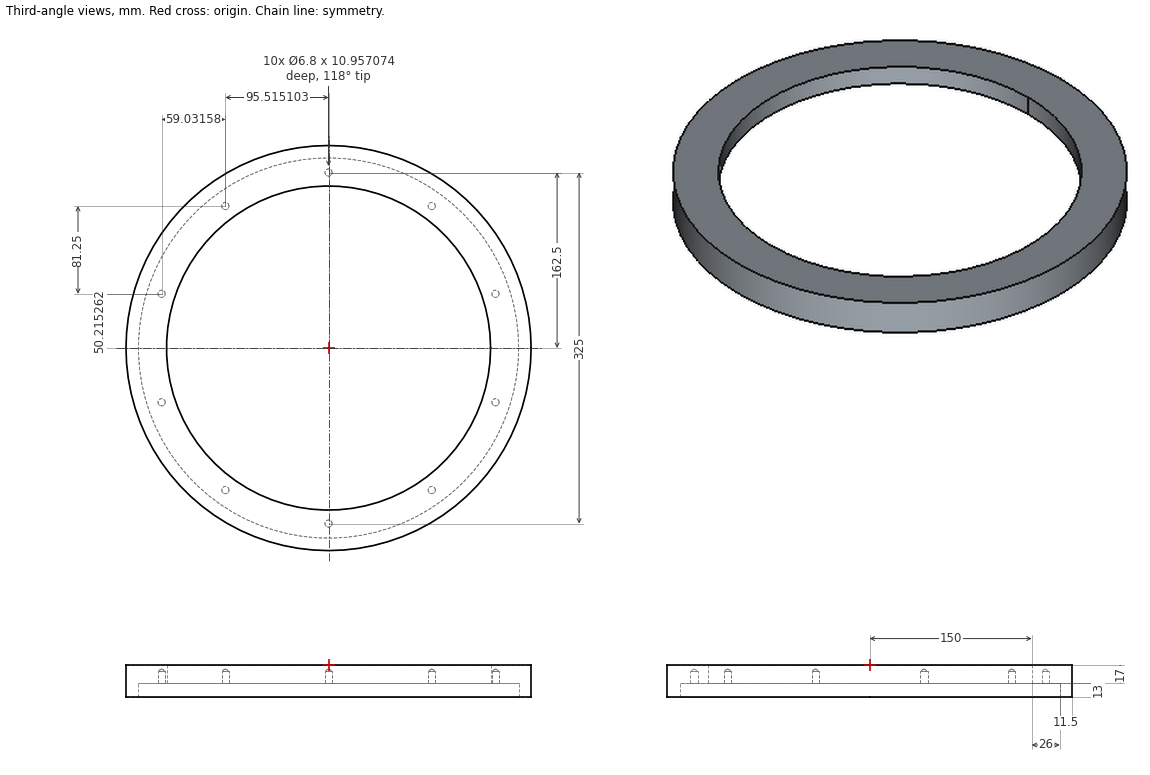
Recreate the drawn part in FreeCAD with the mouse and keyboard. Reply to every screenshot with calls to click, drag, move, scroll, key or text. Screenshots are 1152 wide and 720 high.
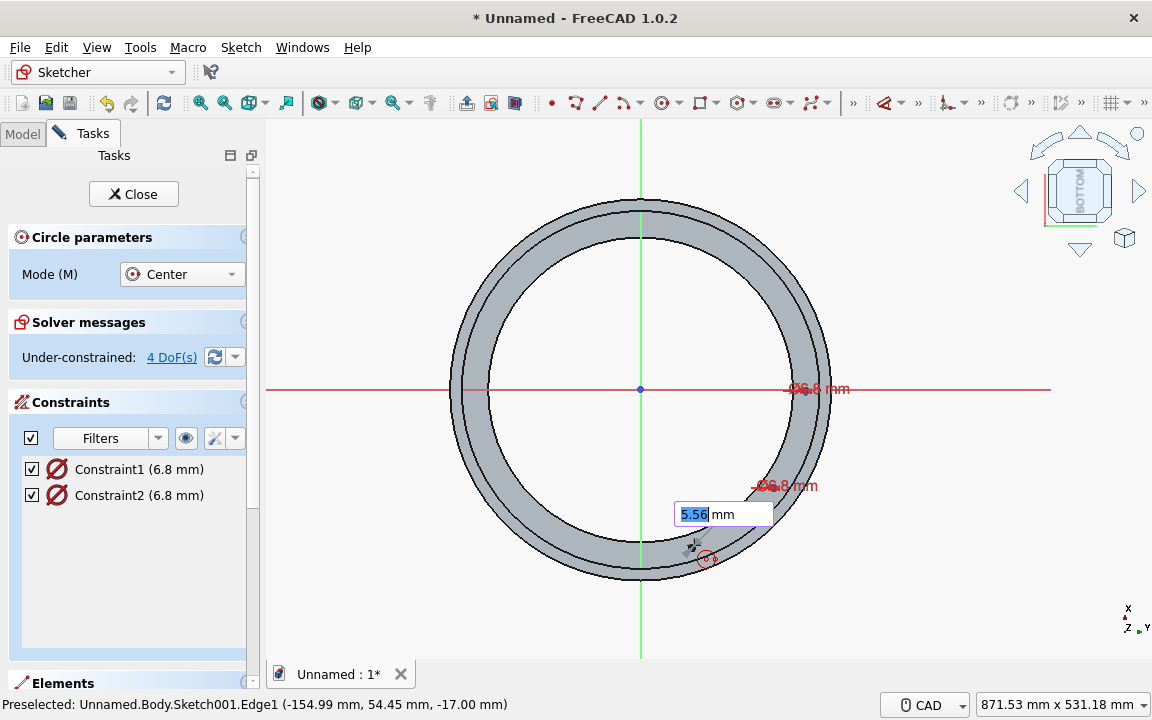
text(6.8)
key(Return)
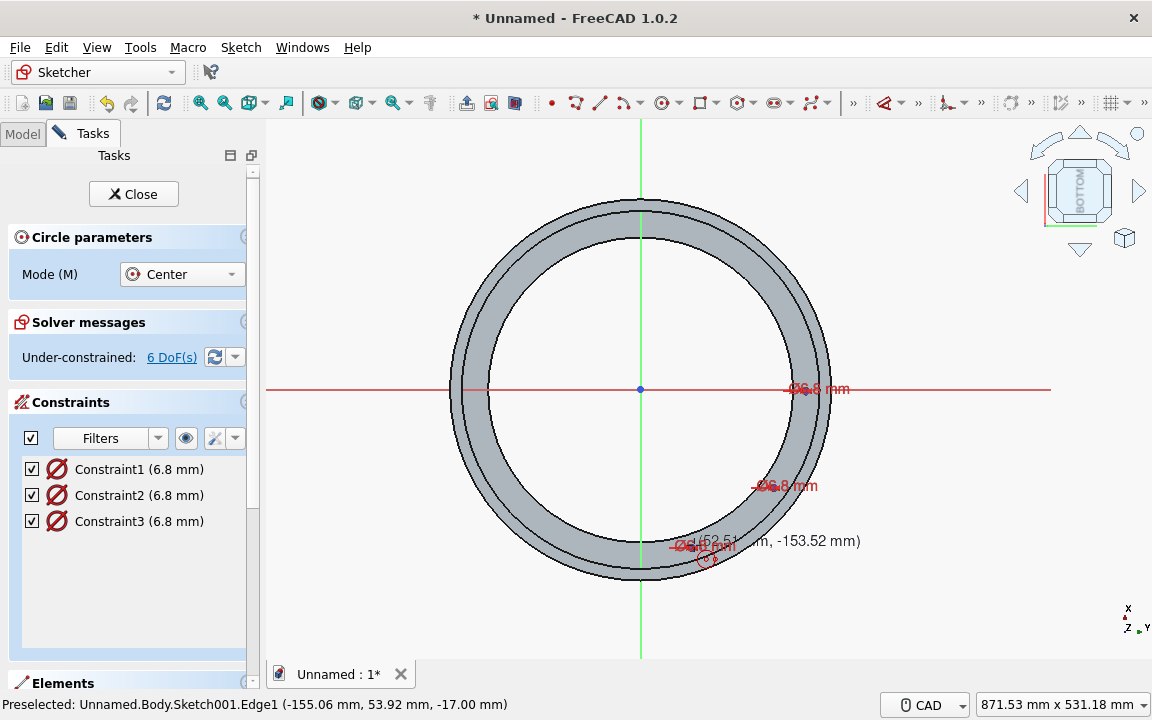
scroll(590, 547, up, 10)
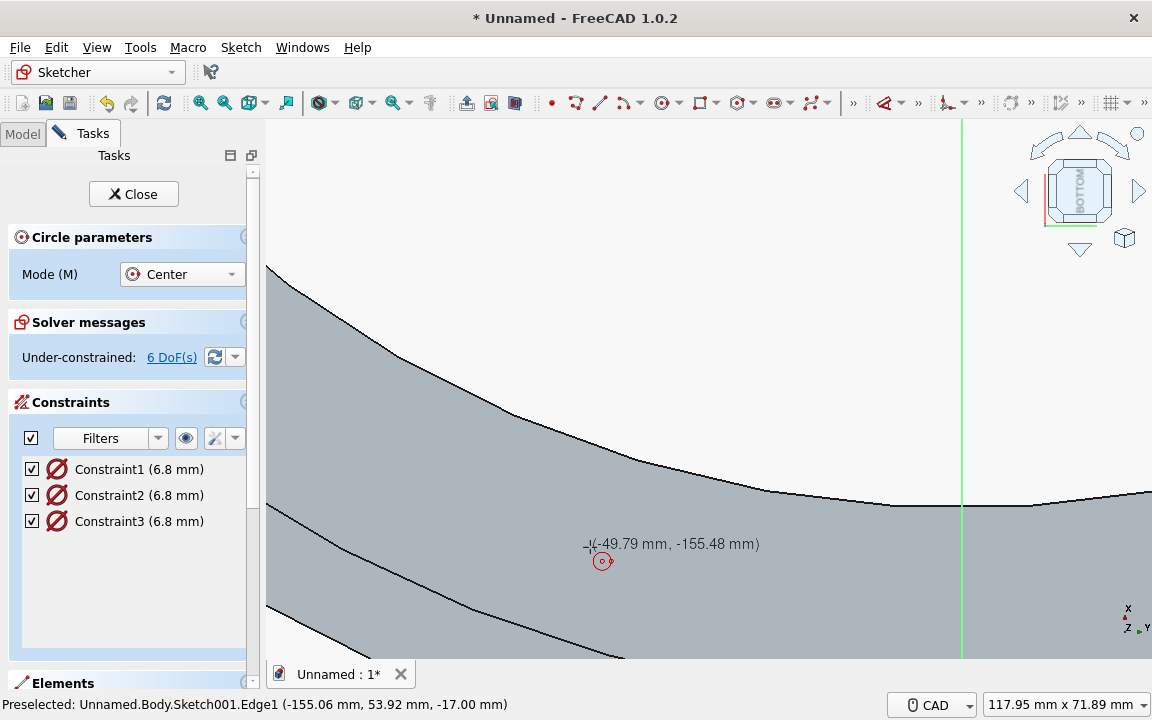
scroll(590, 547, down, 10)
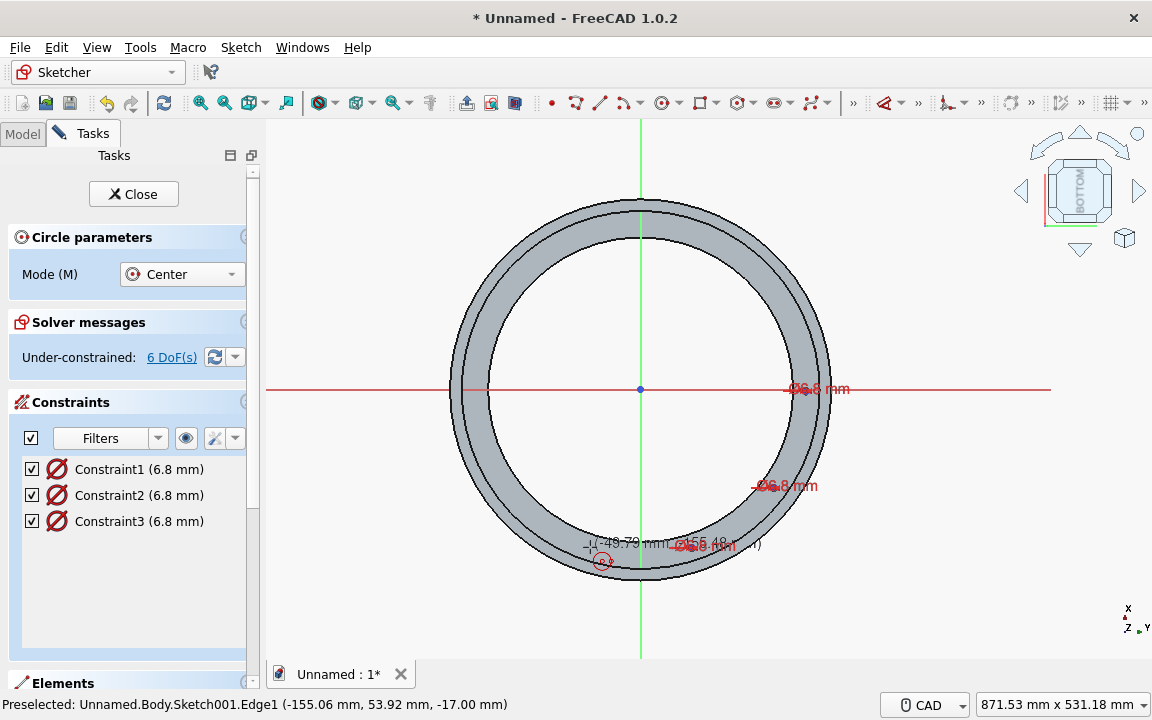
click(590, 547)
move(592, 545)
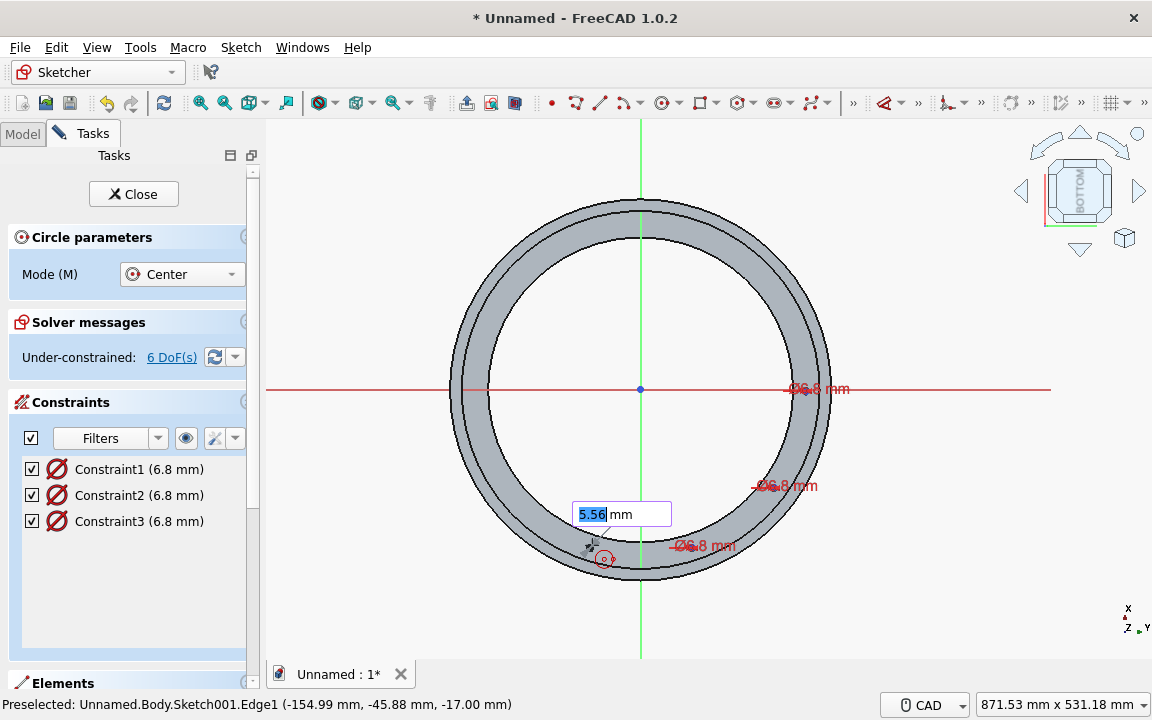
text(6.8)
key(Return)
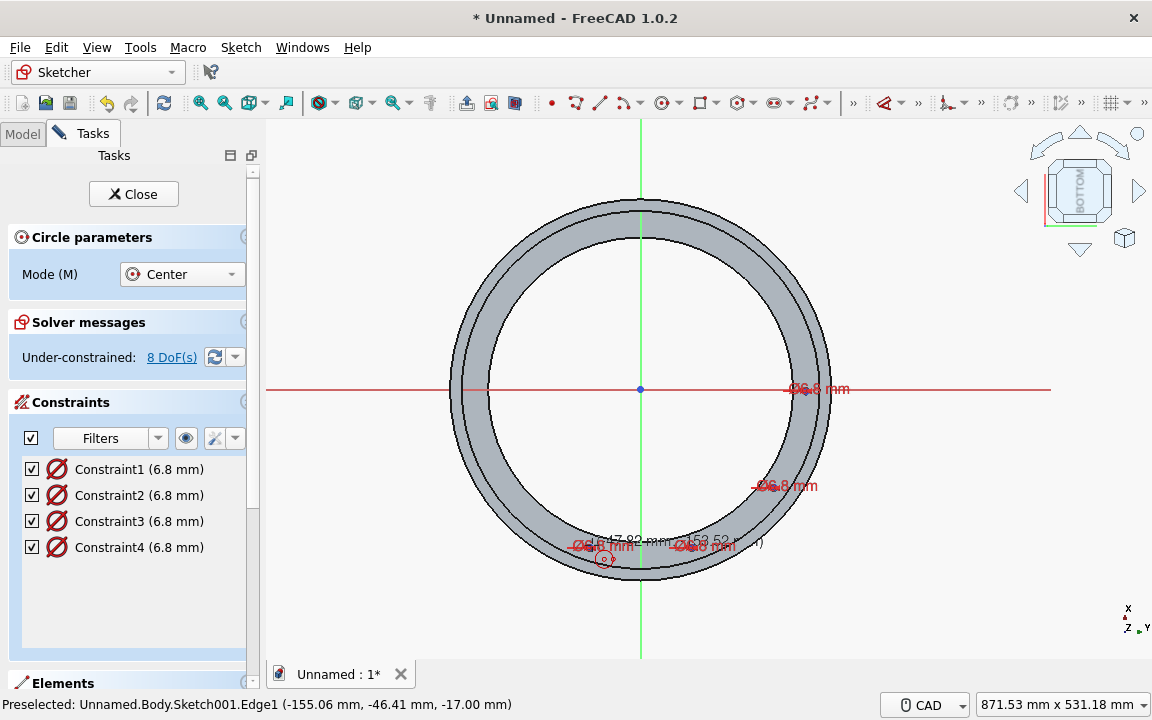
scroll(507, 487, up, 10)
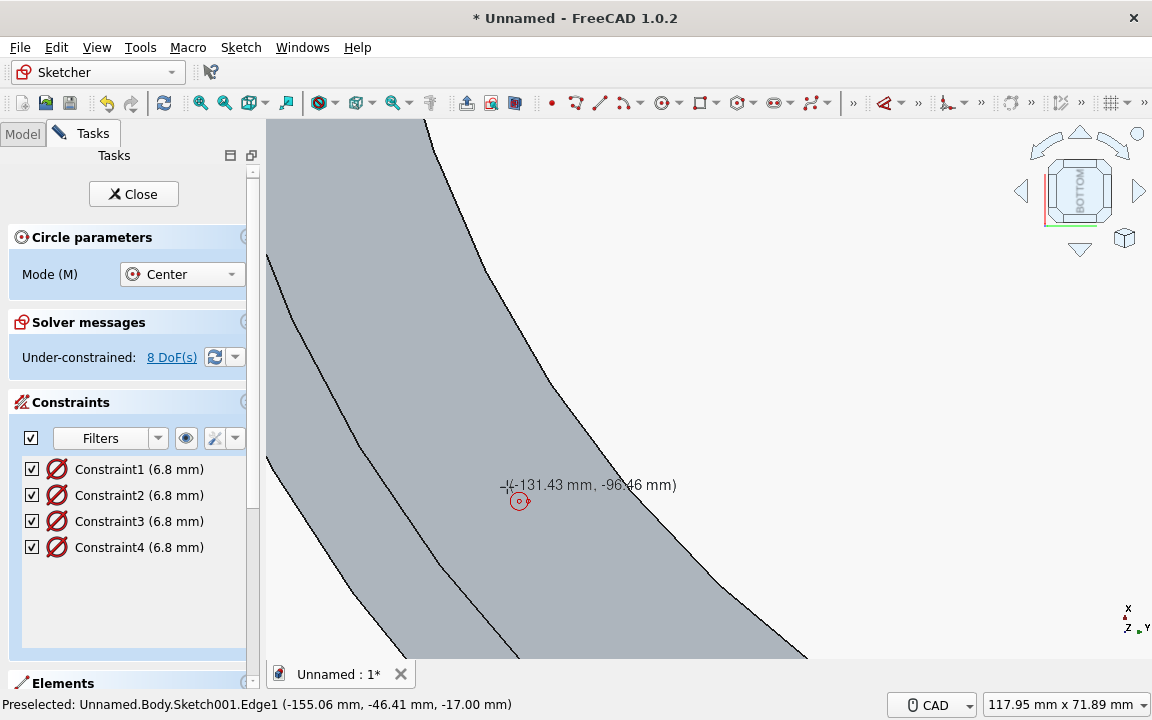
scroll(507, 487, down, 10)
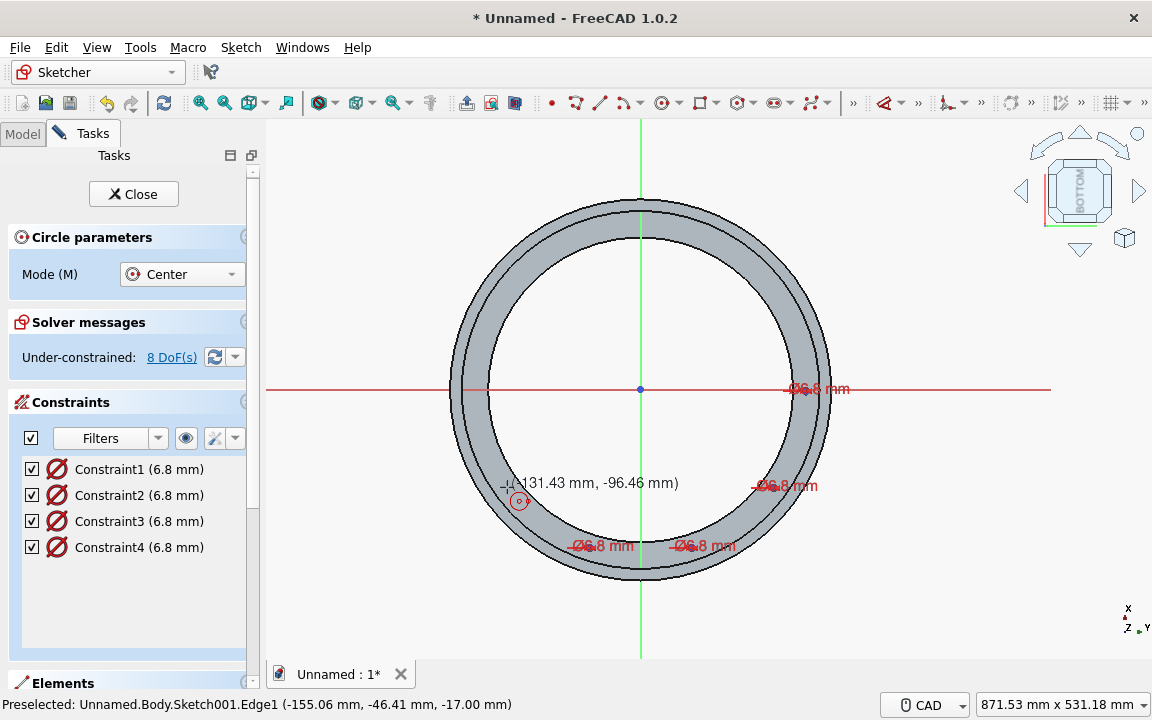
click(507, 487)
move(509, 485)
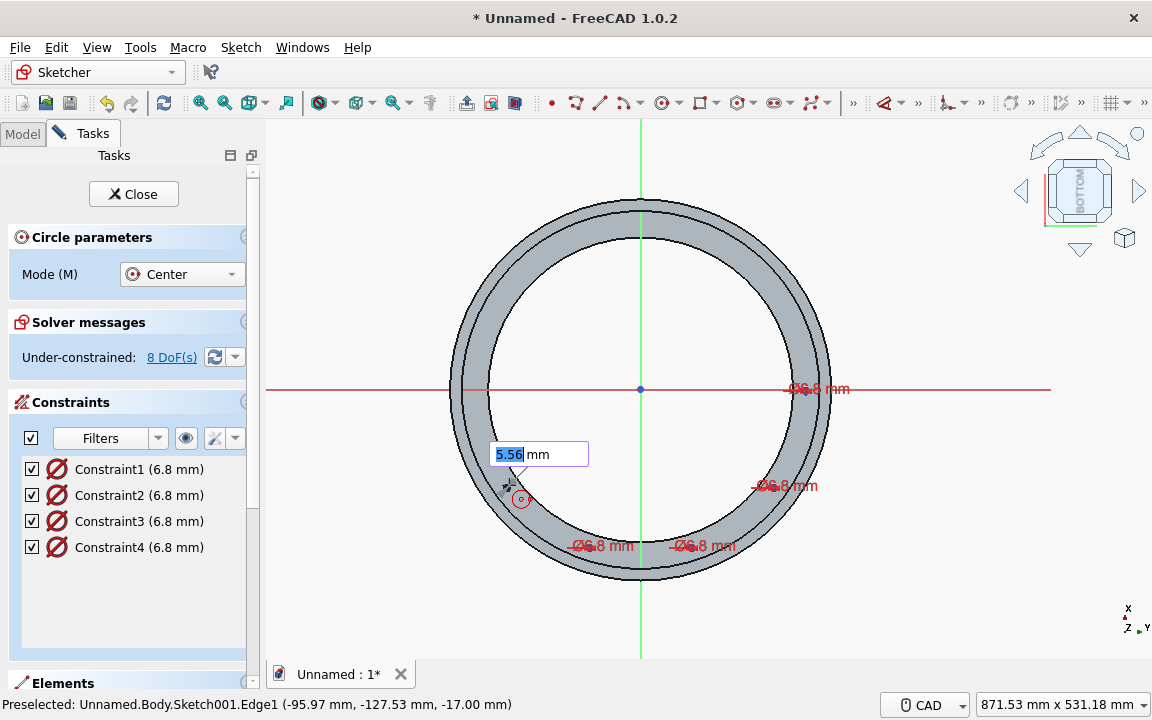
text(6.8)
key(Return)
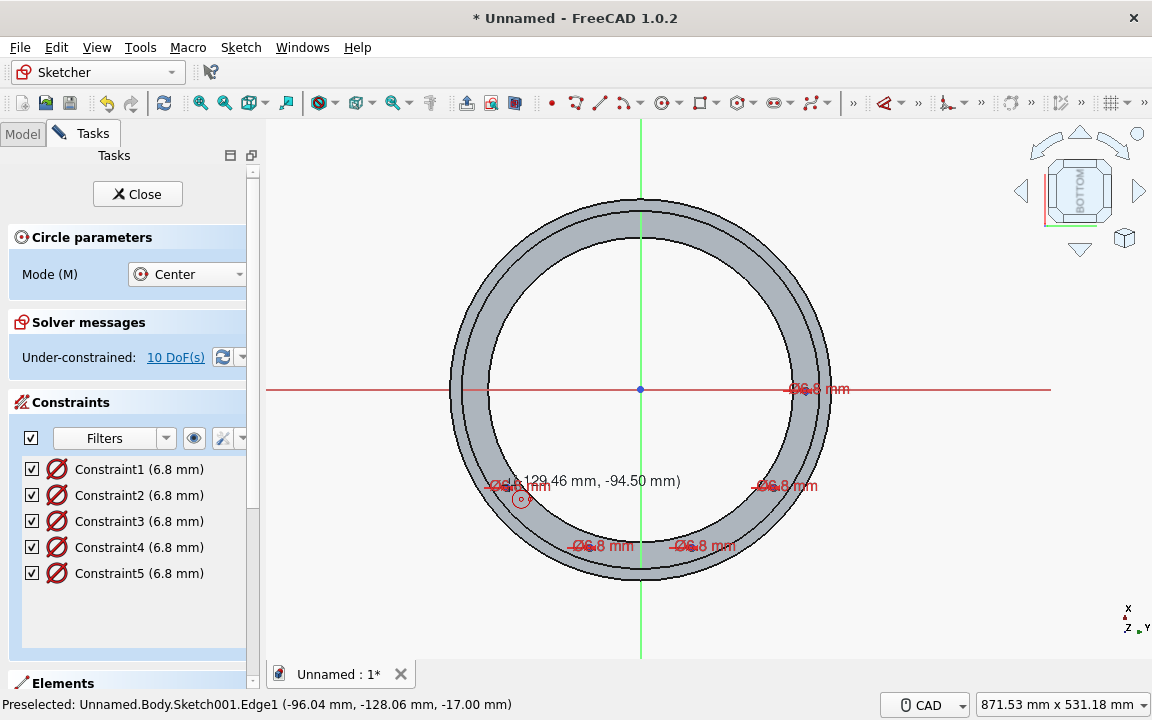
scroll(475, 390, up, 10)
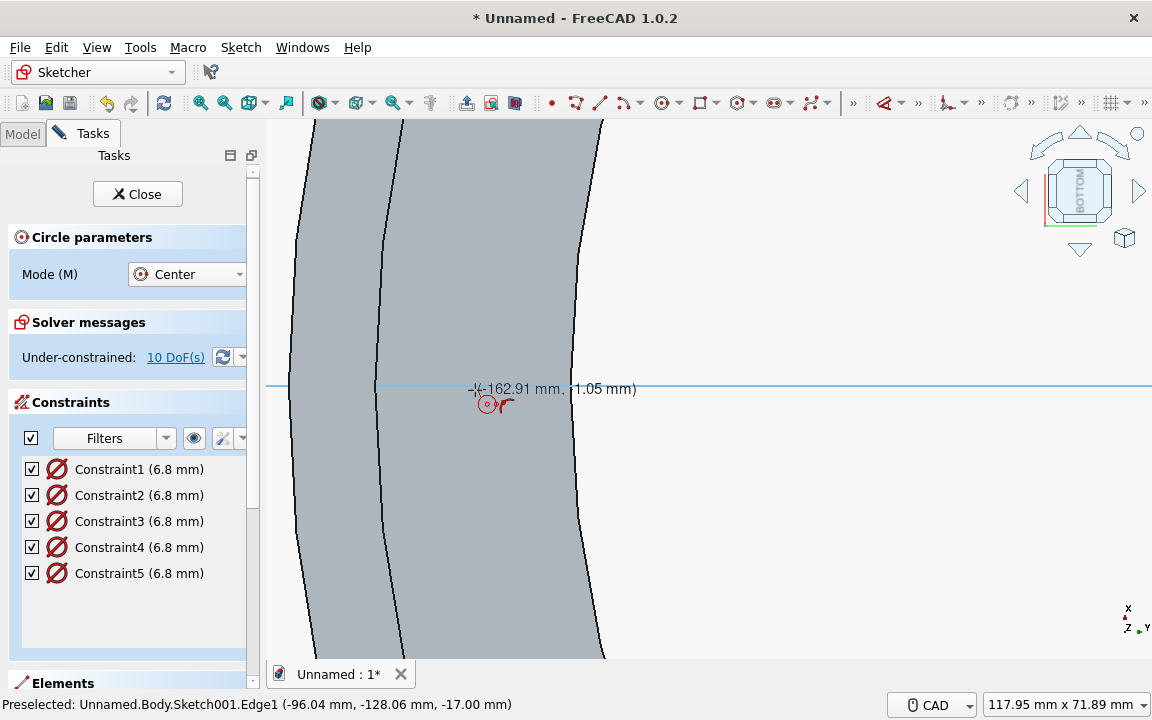
scroll(475, 389, down, 10)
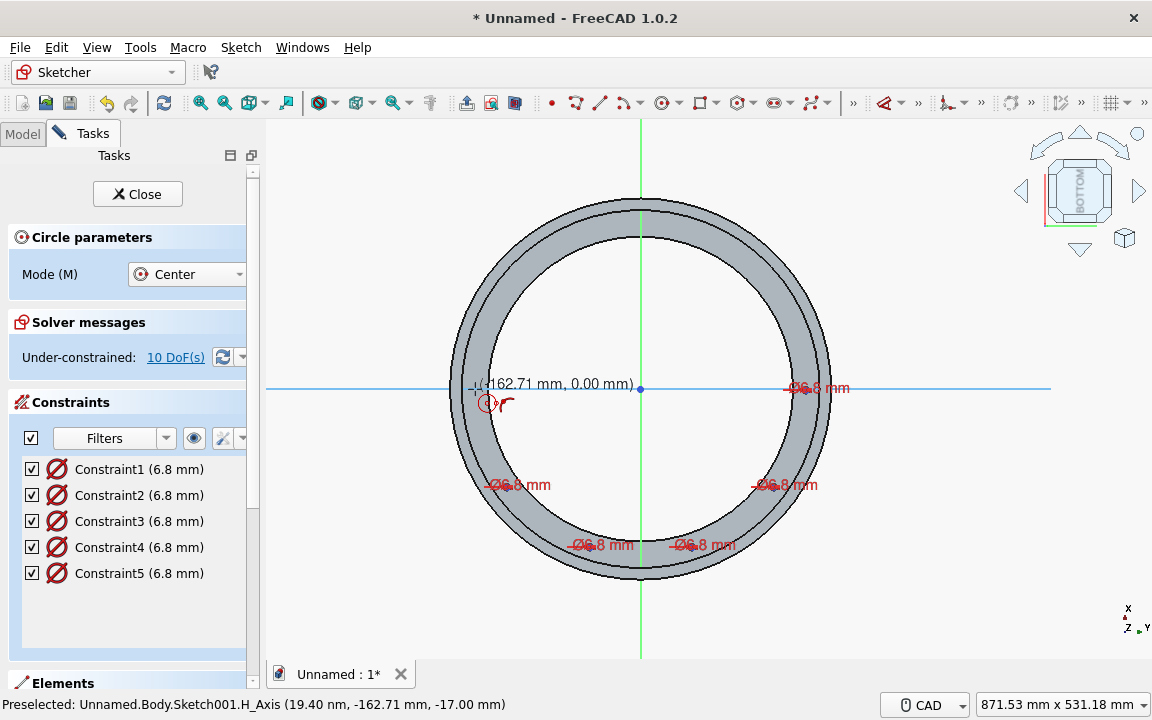
click(475, 389)